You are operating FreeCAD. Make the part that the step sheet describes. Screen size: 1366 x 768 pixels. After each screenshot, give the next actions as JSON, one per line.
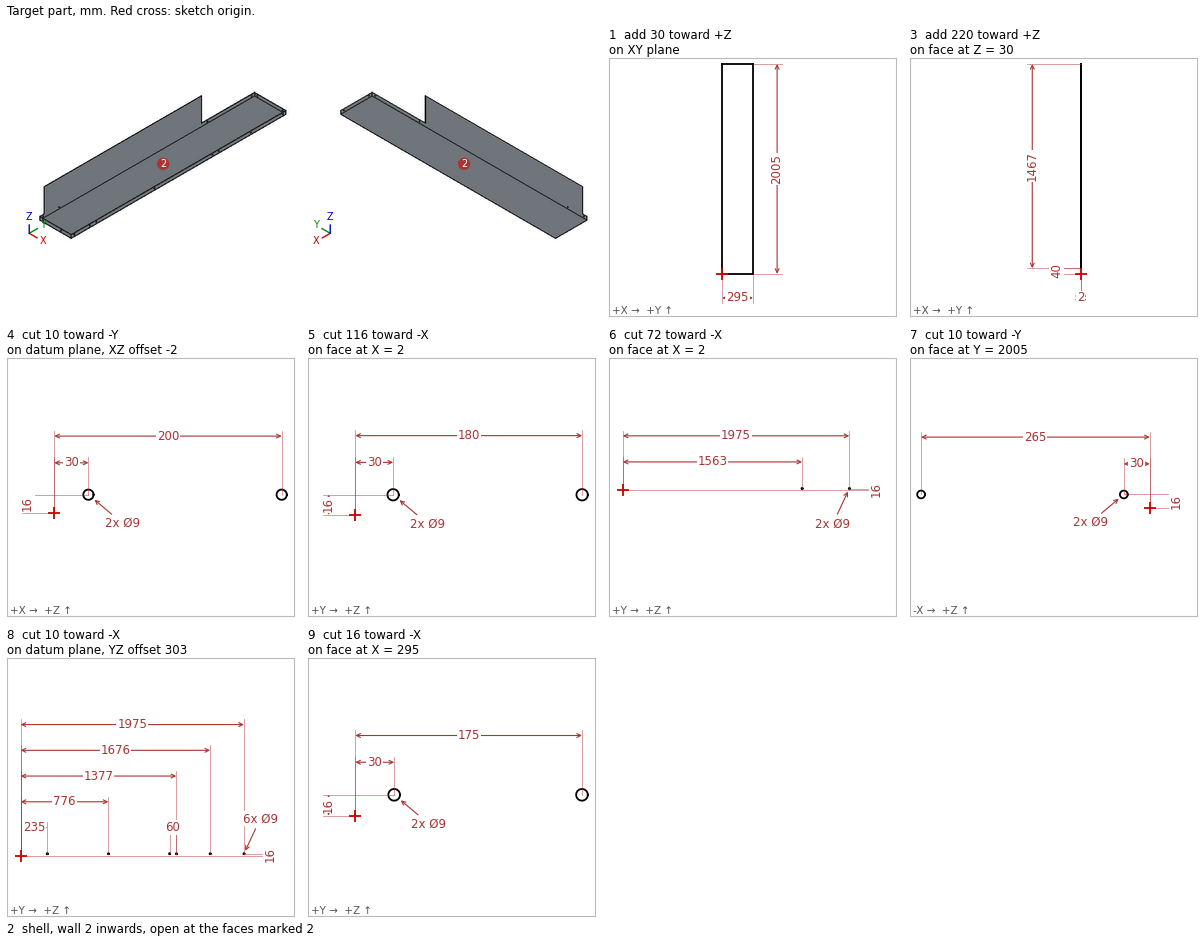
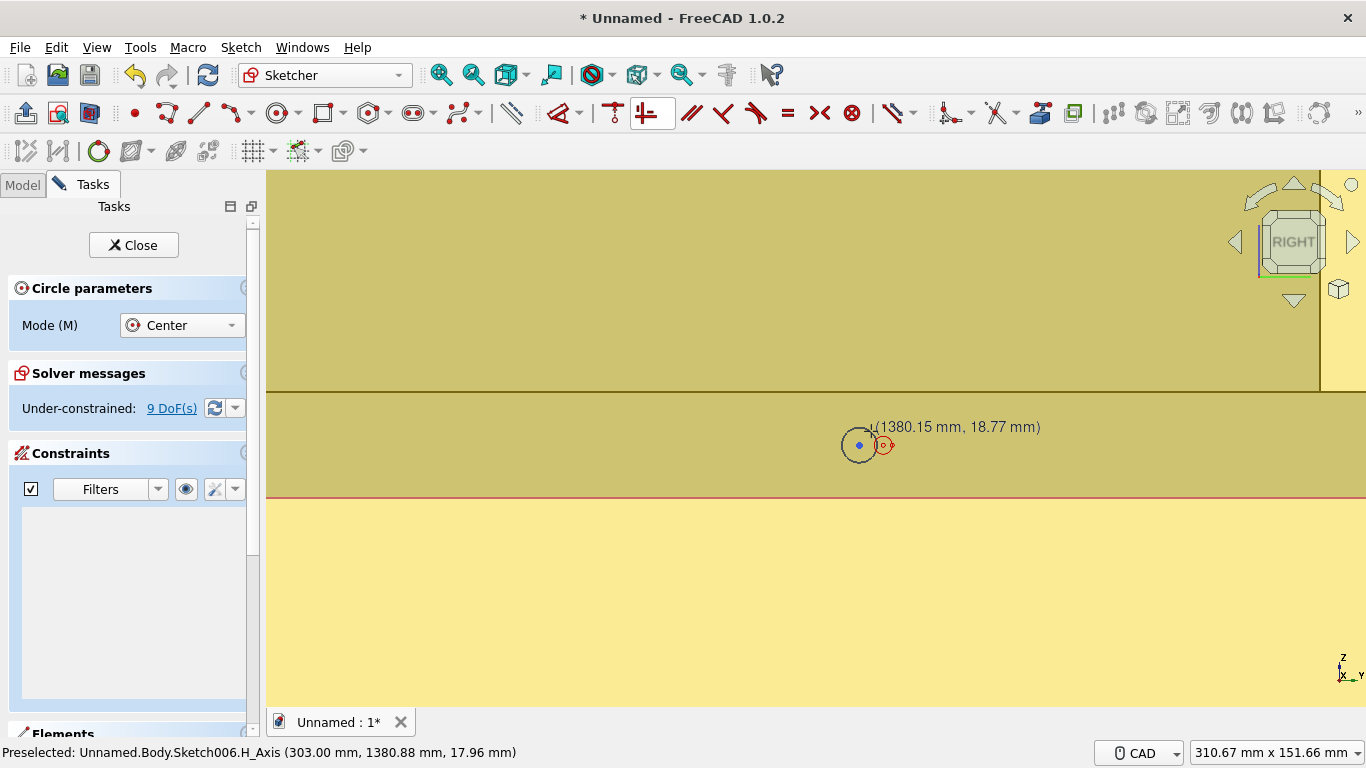
{"action": "scroll", "coordinate": [647, 442], "scroll_direction": "up", "scroll_amount": 2}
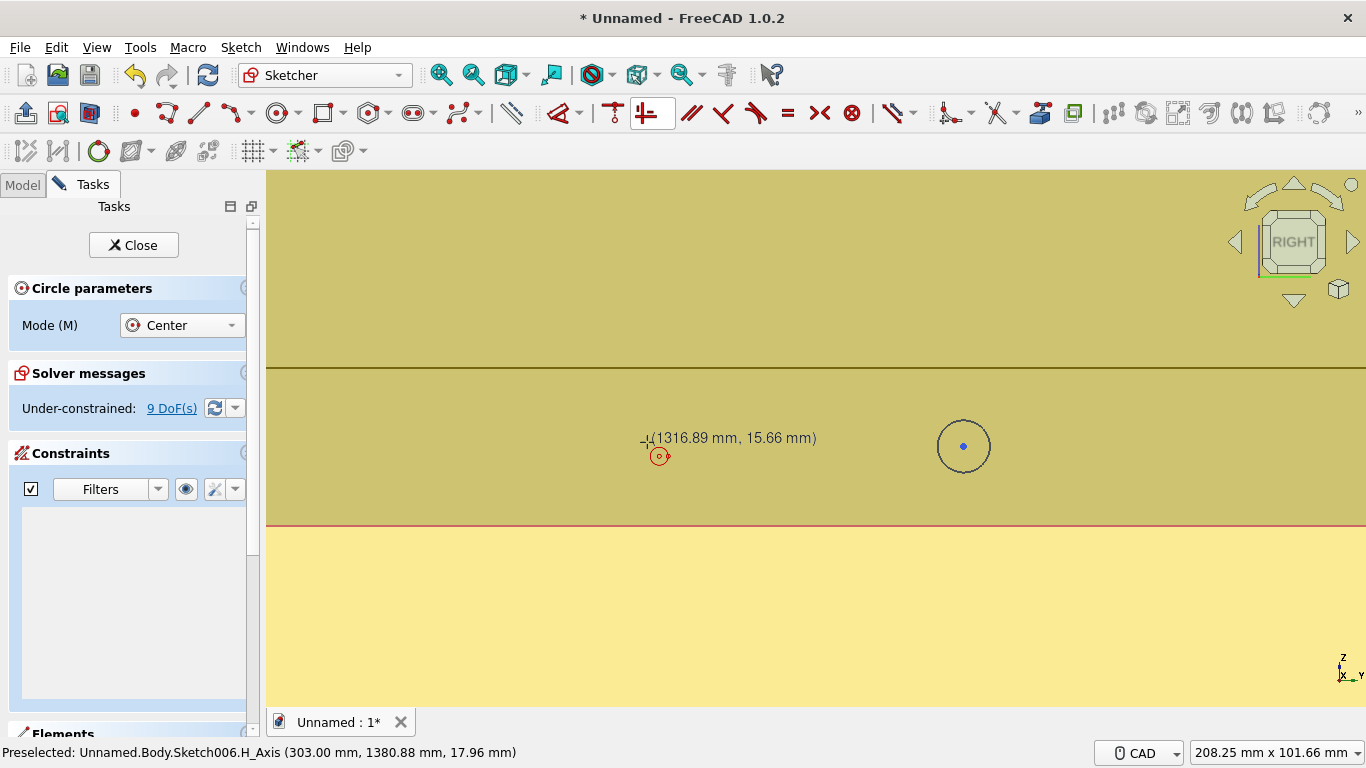
{"action": "scroll", "coordinate": [866, 436], "scroll_direction": "down", "scroll_amount": 14}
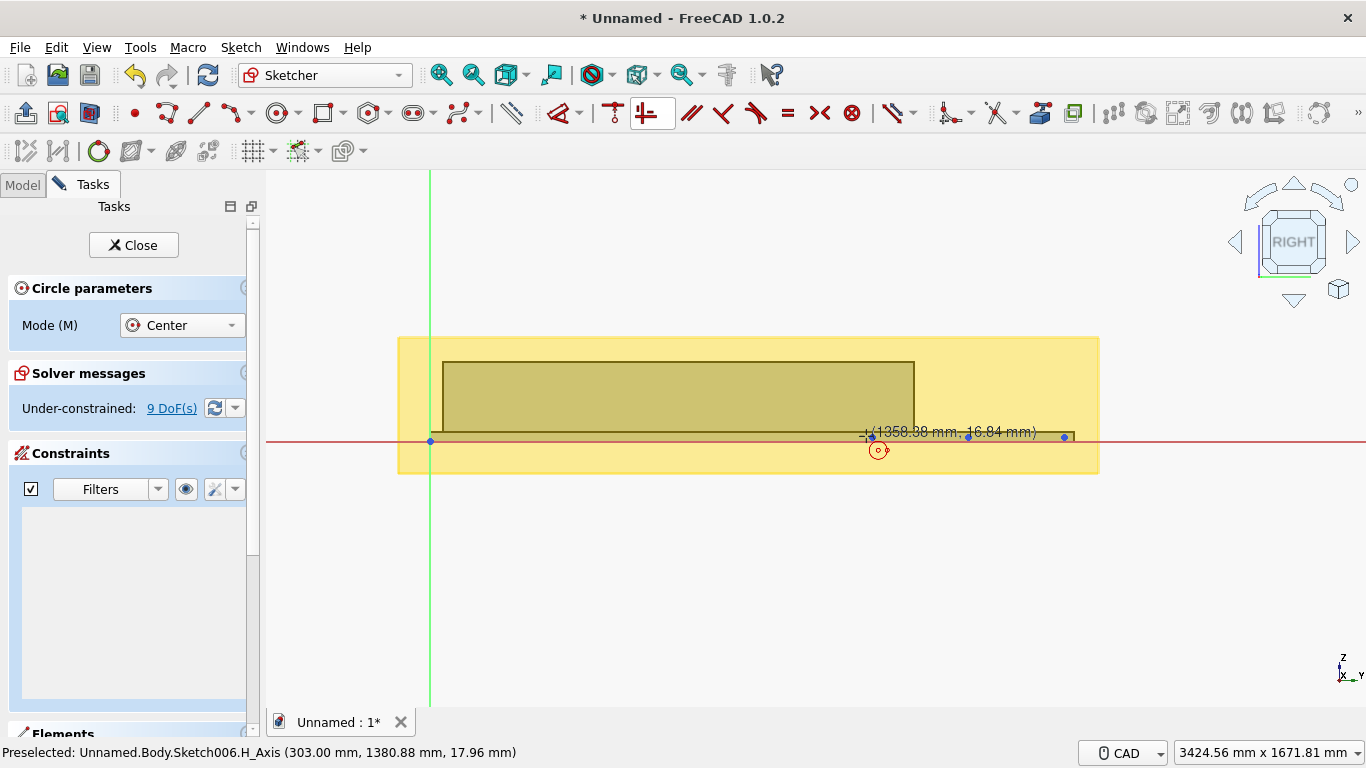
{"action": "scroll", "coordinate": [853, 437], "scroll_direction": "up", "scroll_amount": 6}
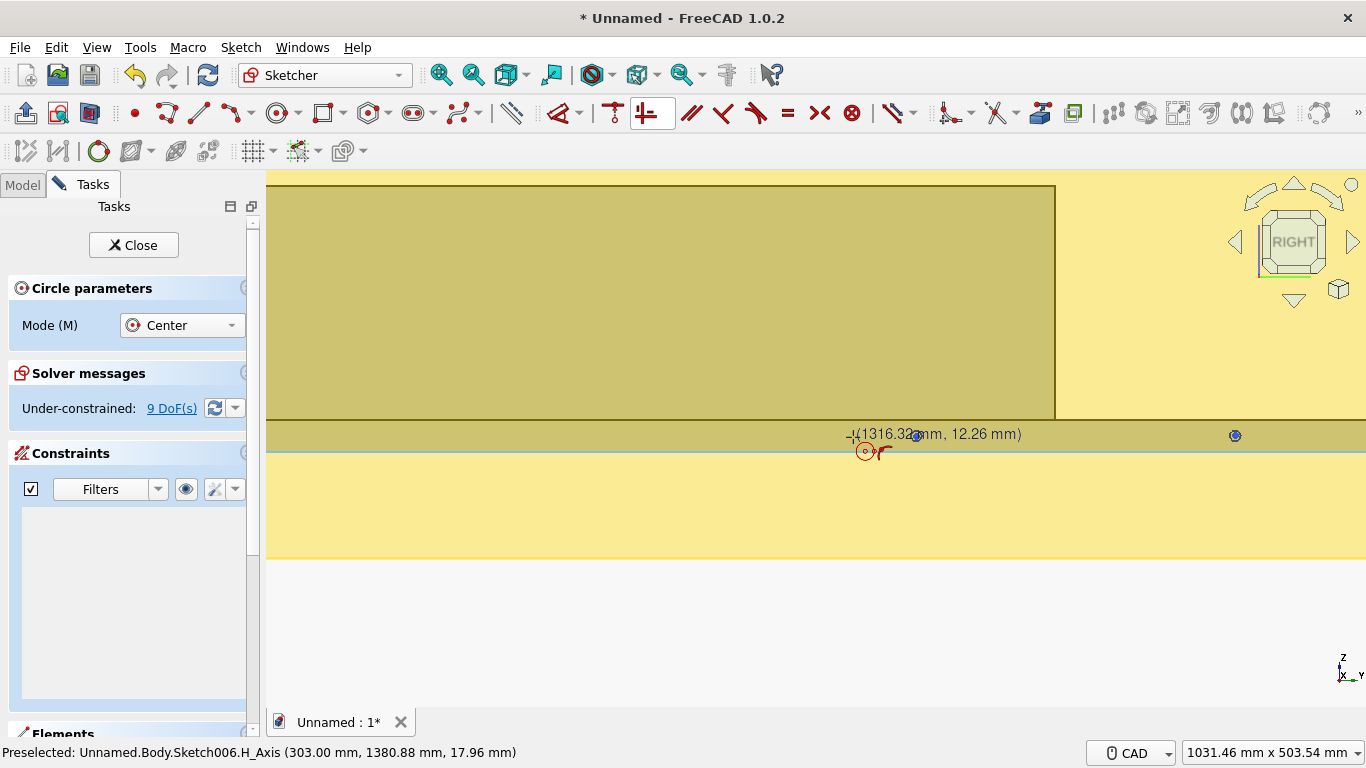
{"action": "left_click", "coordinate": [852, 435]}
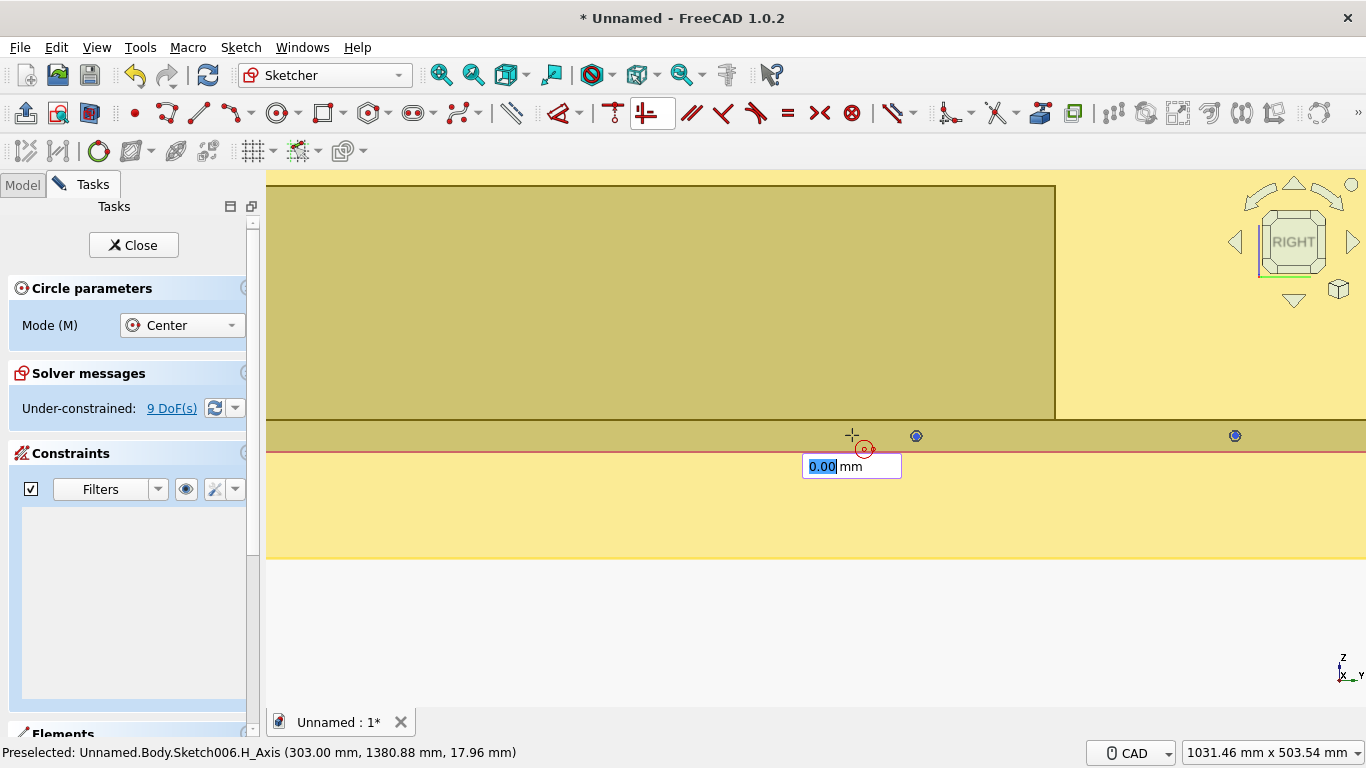
{"action": "scroll", "coordinate": [856, 432], "scroll_direction": "up", "scroll_amount": 6}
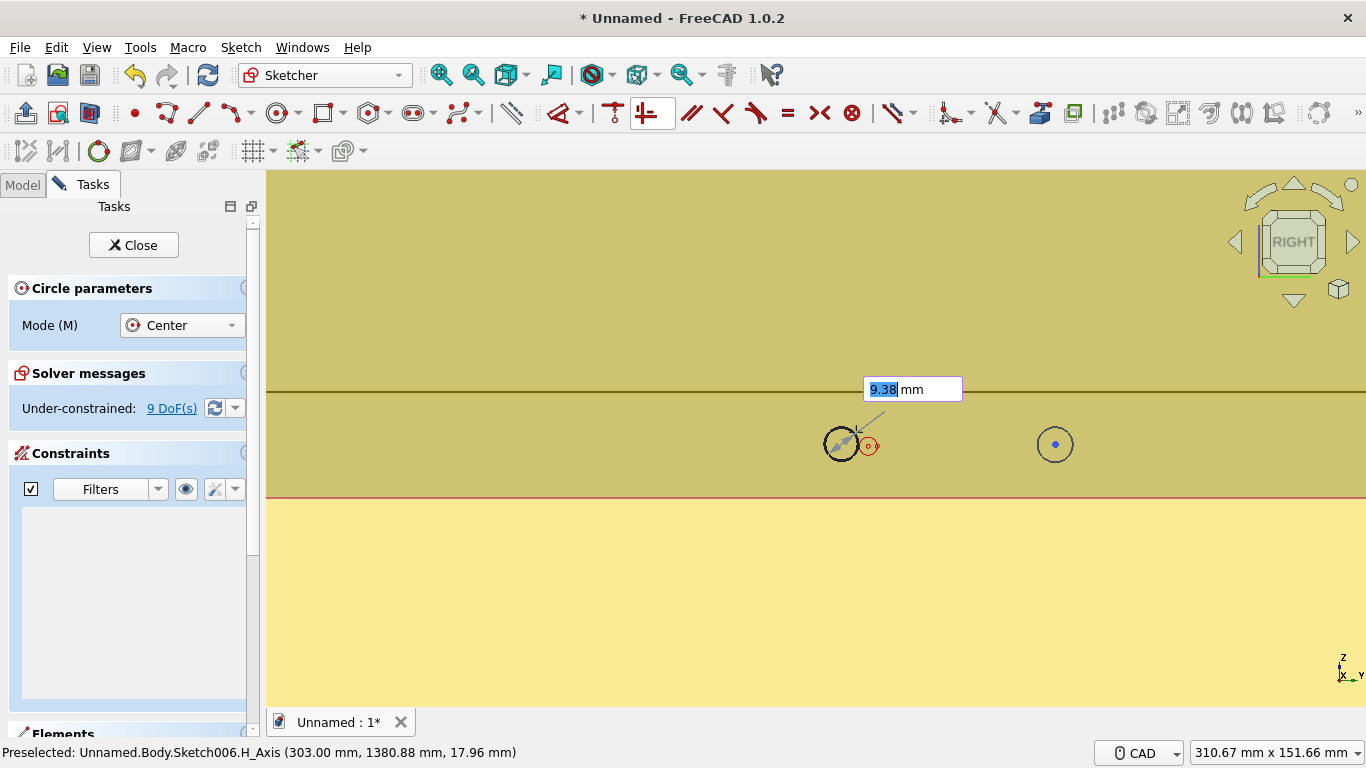
{"action": "left_click", "coordinate": [854, 430]}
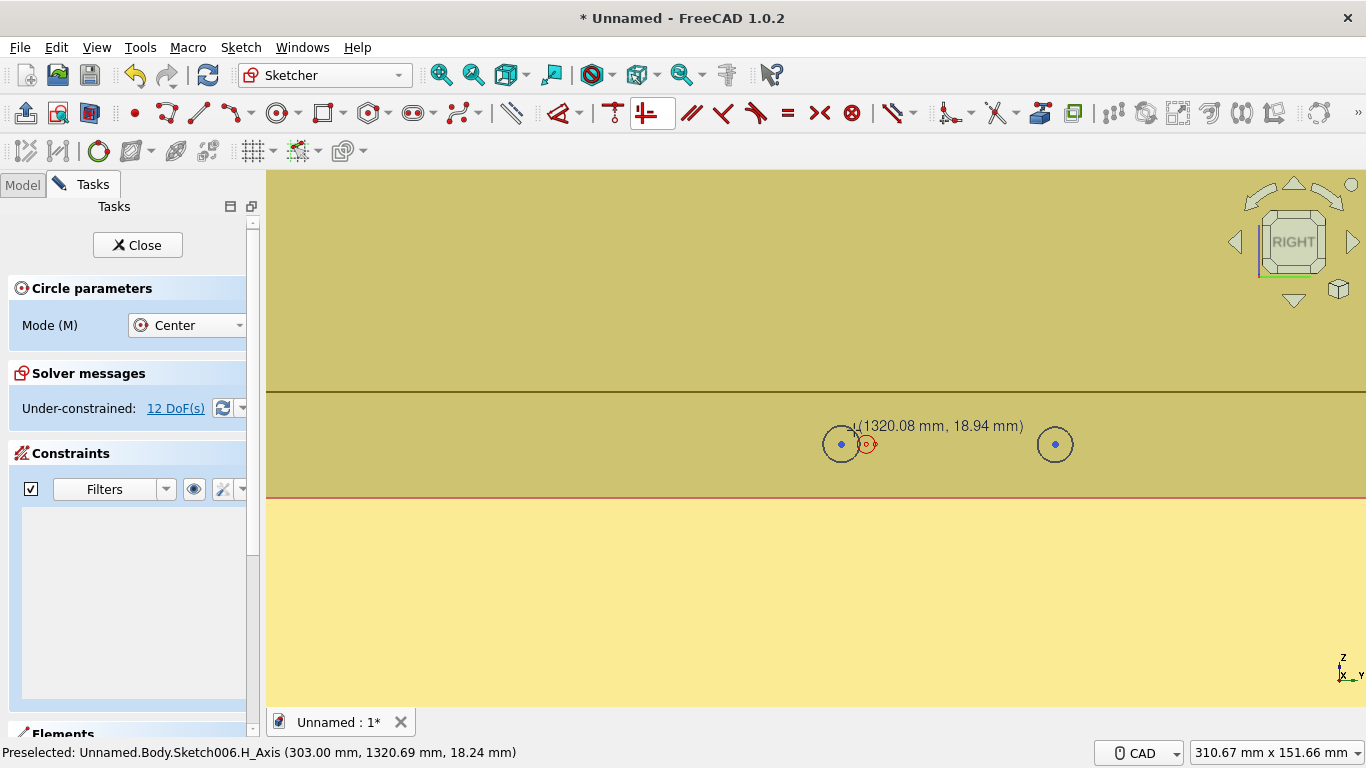
{"action": "scroll", "coordinate": [854, 436], "scroll_direction": "down", "scroll_amount": 12}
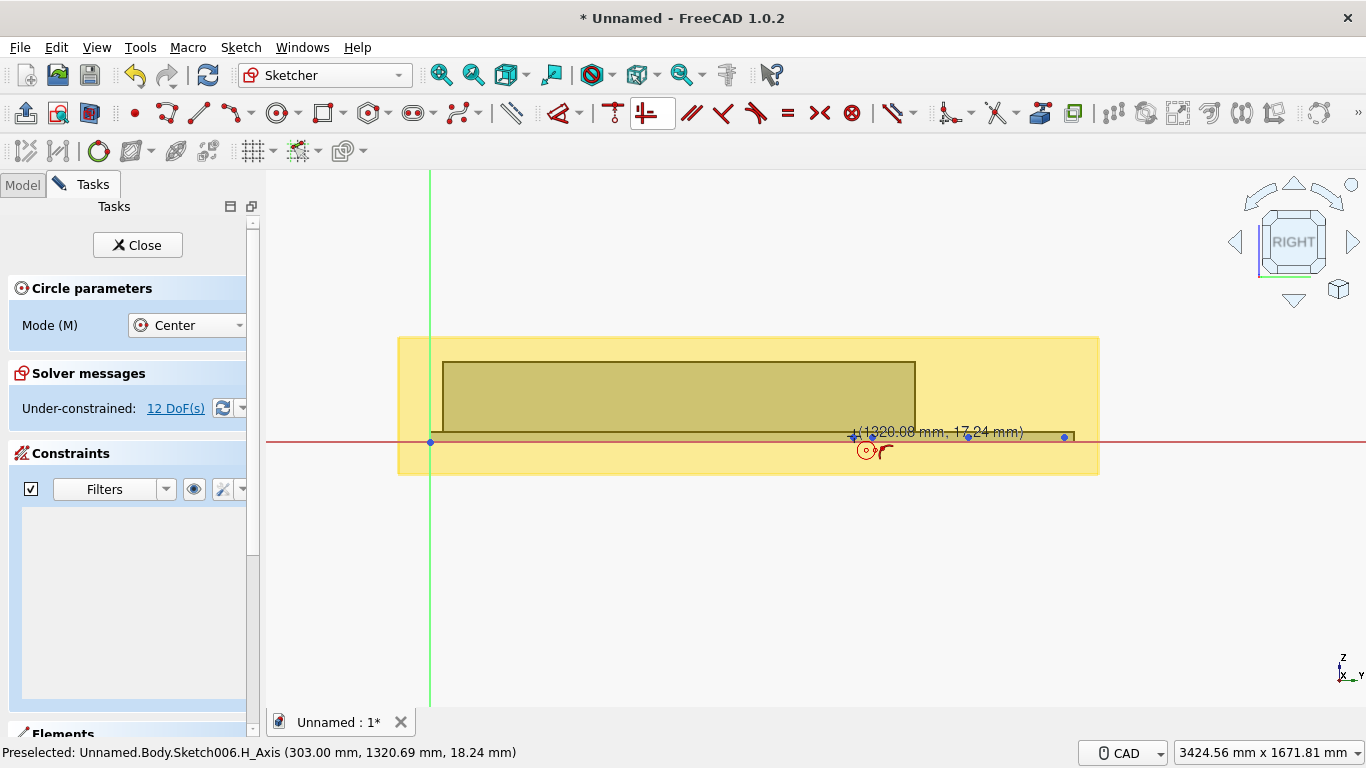
{"action": "scroll", "coordinate": [680, 437], "scroll_direction": "up", "scroll_amount": 14}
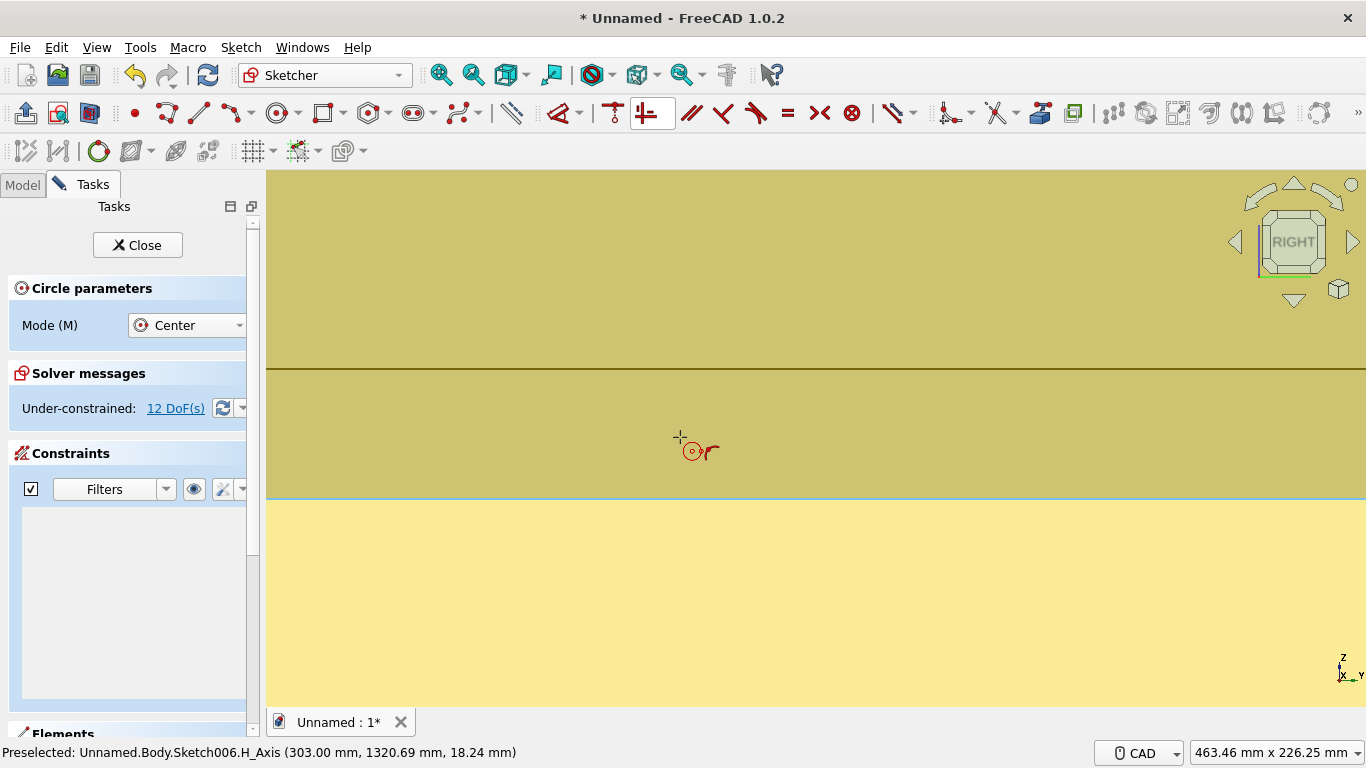
{"action": "scroll", "coordinate": [679, 437], "scroll_direction": "down", "scroll_amount": 14}